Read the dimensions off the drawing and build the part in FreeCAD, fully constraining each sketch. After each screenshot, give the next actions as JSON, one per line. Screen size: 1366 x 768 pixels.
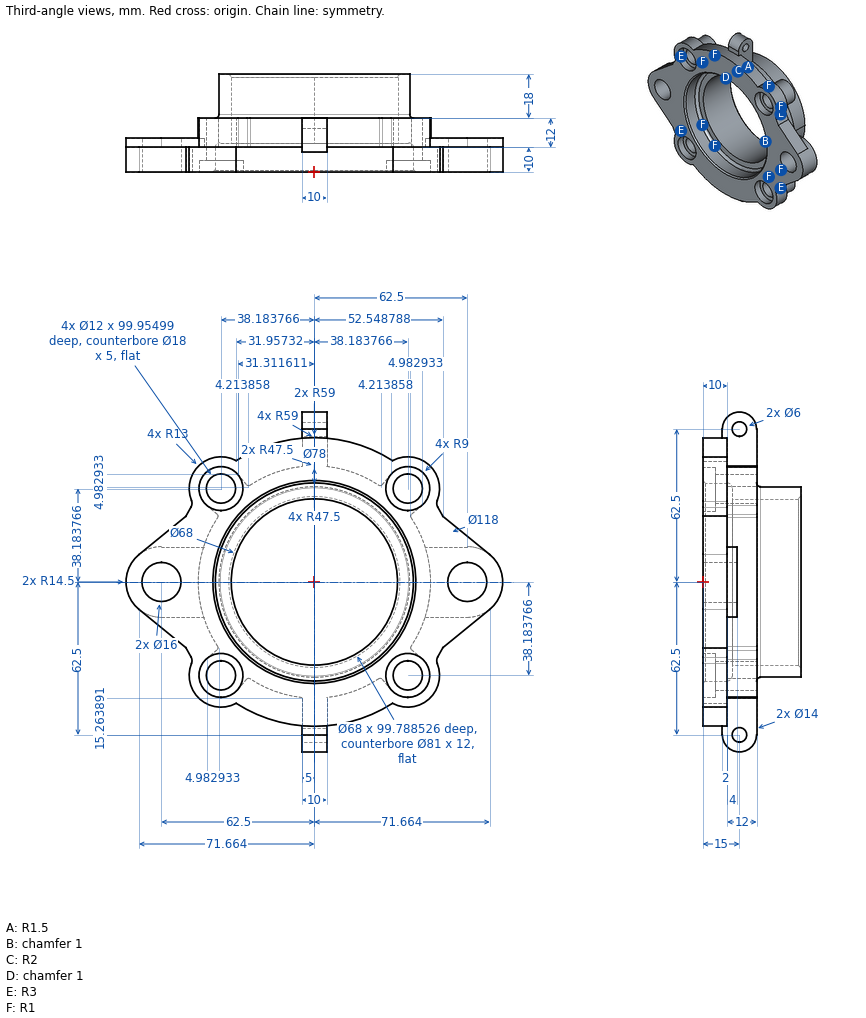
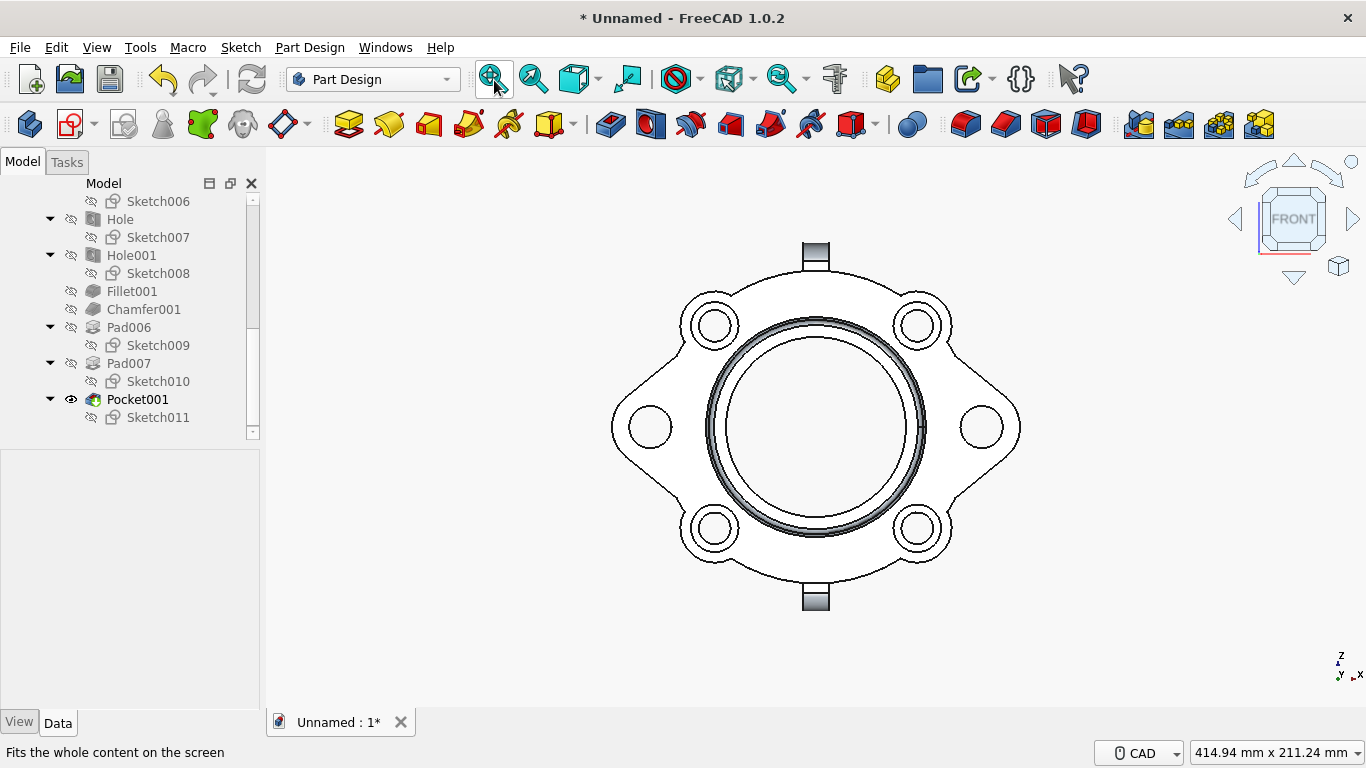
{"action": "key", "text": "3"}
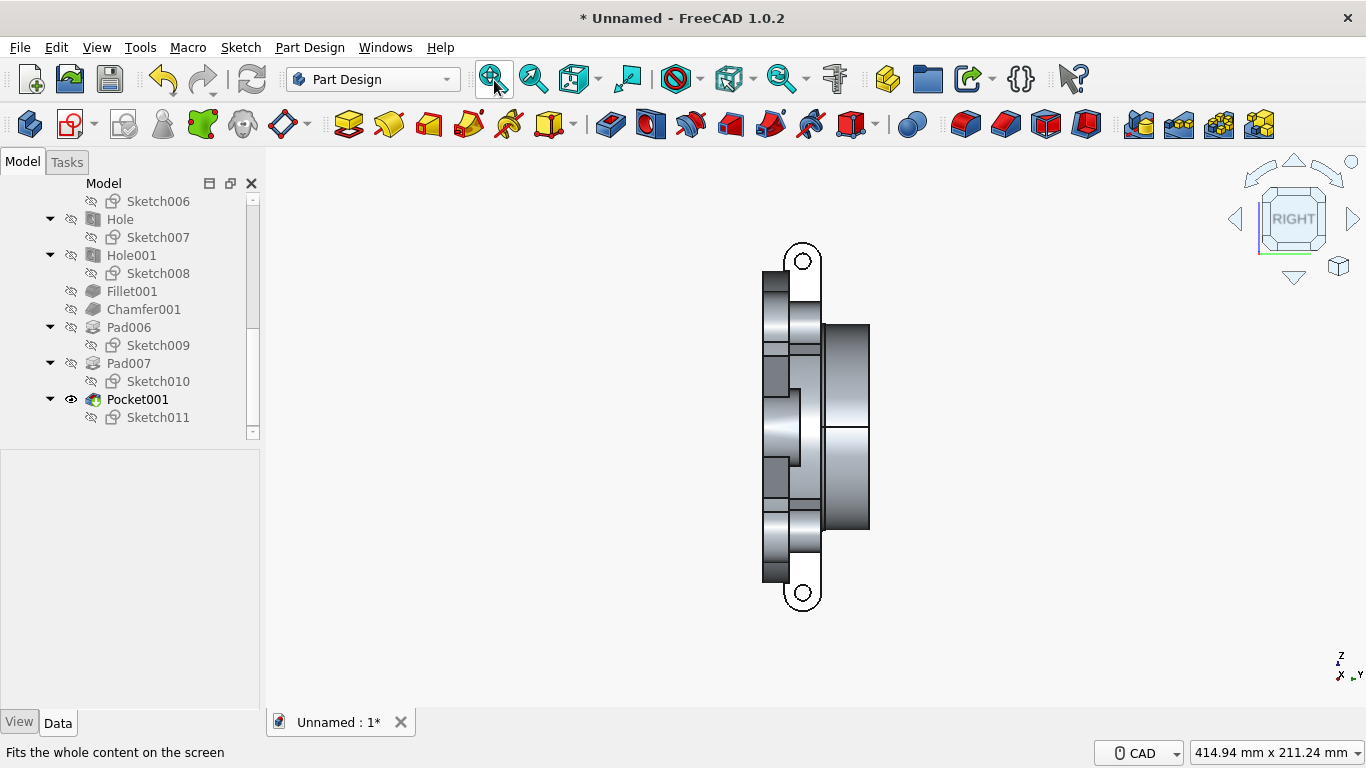
{"action": "key", "text": "5"}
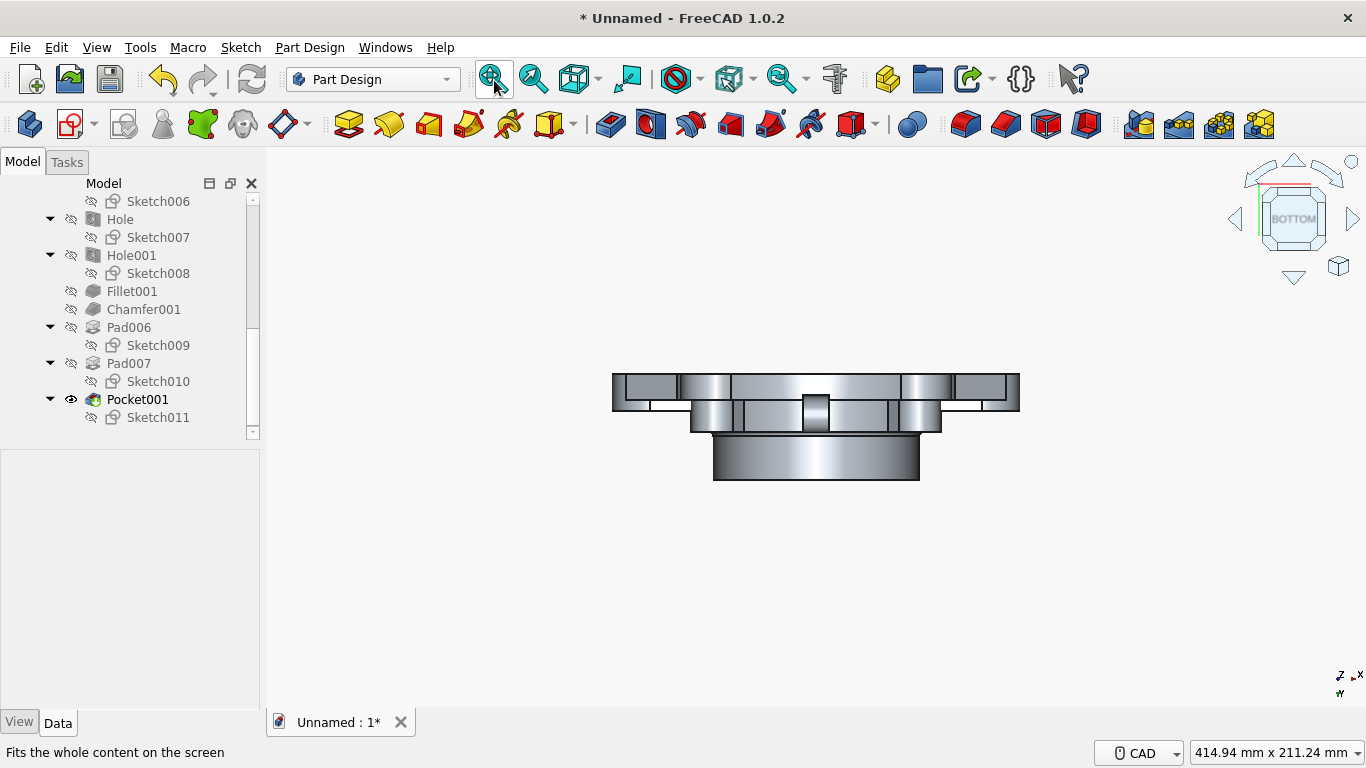
{"action": "left_click", "coordinate": [494, 80]}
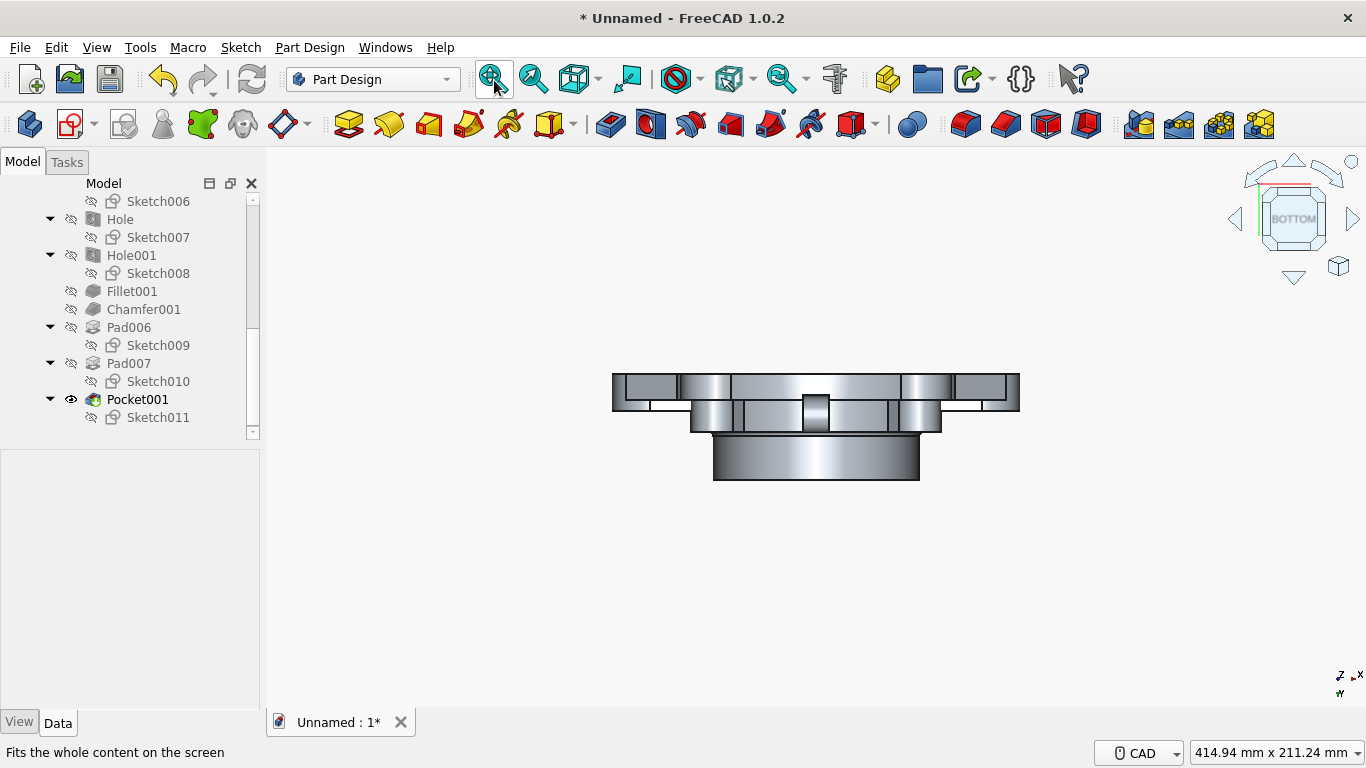
{"action": "key", "text": "4"}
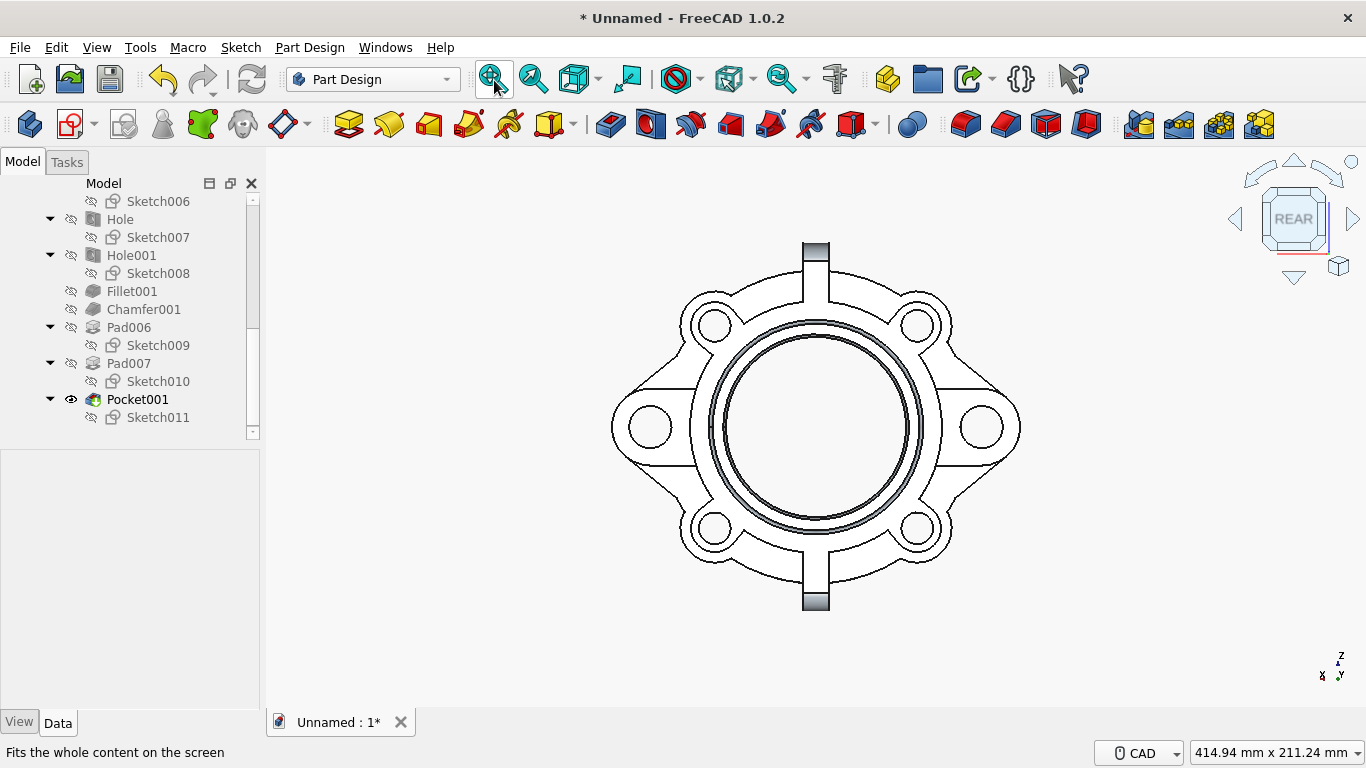
{"action": "key", "text": "6"}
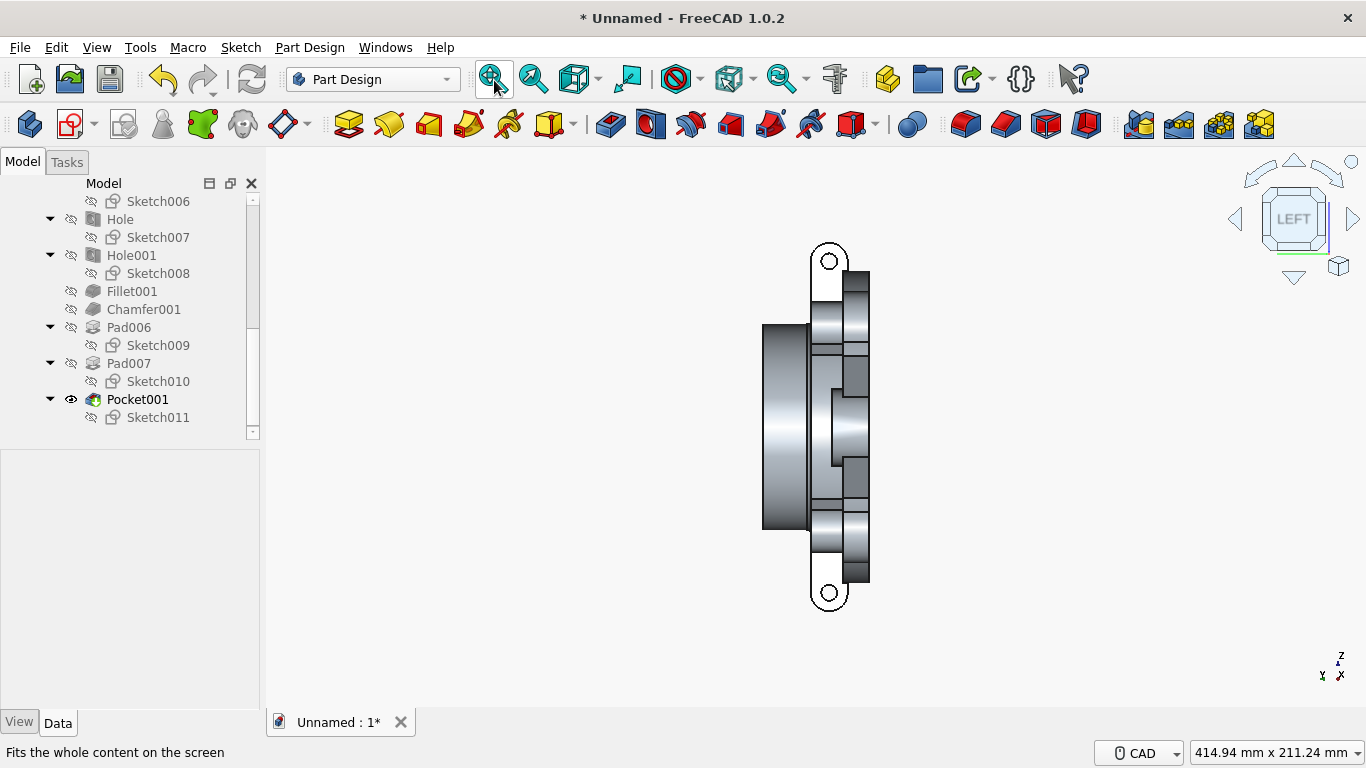
{"action": "key", "text": "v 3"}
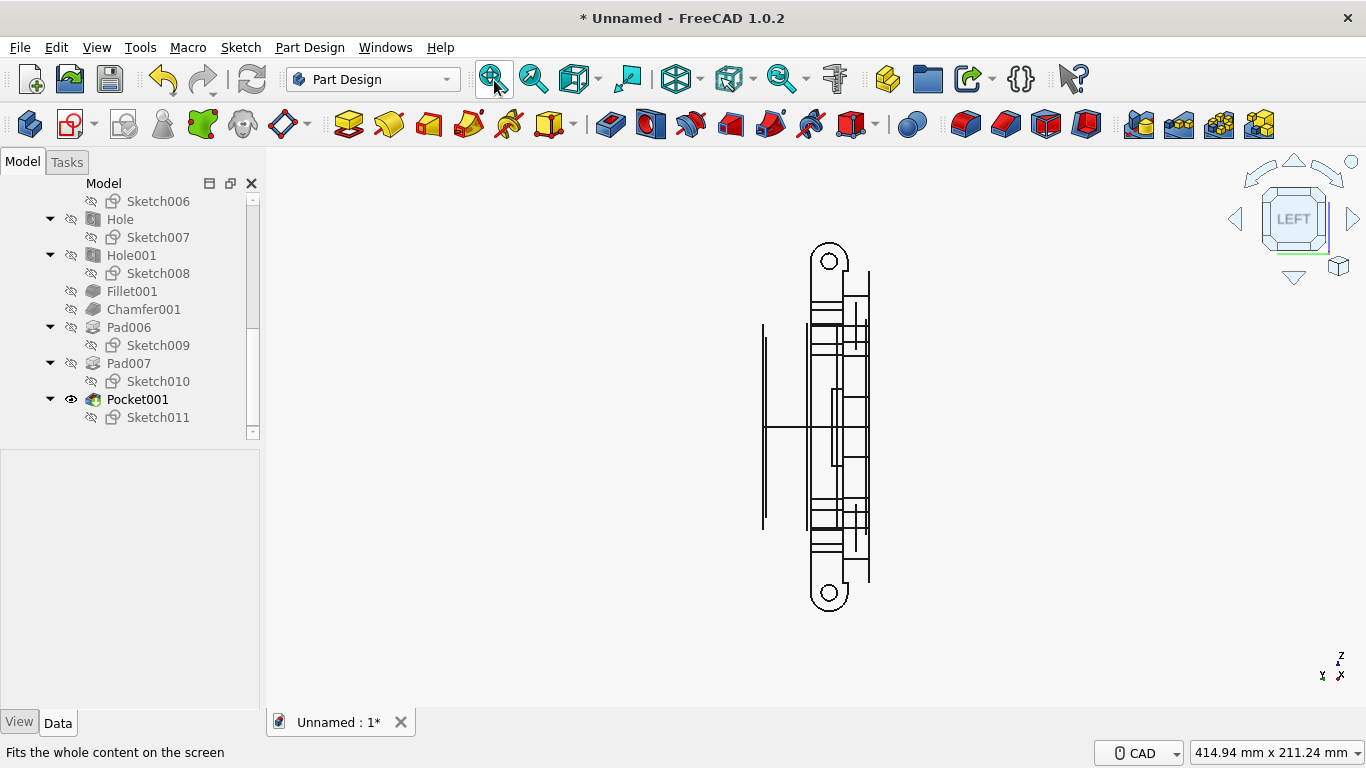
{"action": "key", "text": "0"}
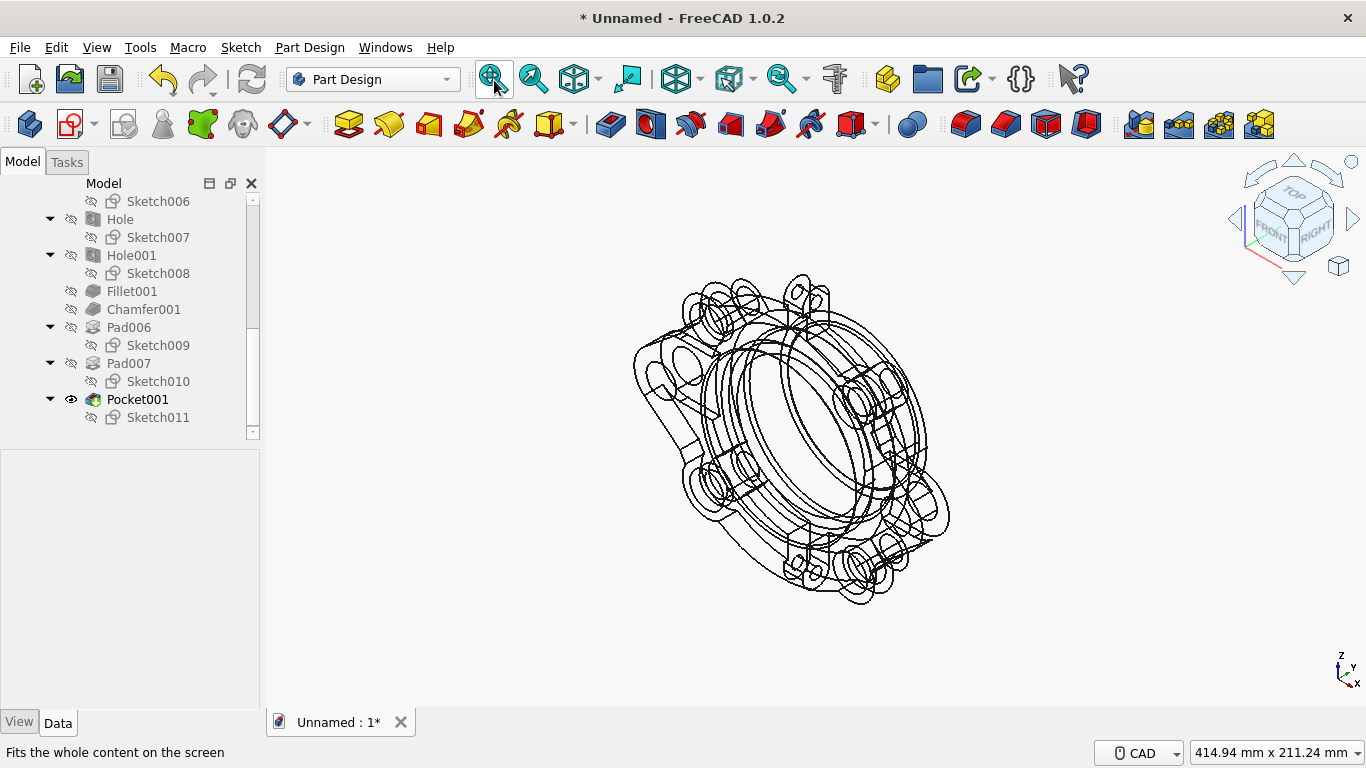
{"action": "left_click", "coordinate": [695, 458]}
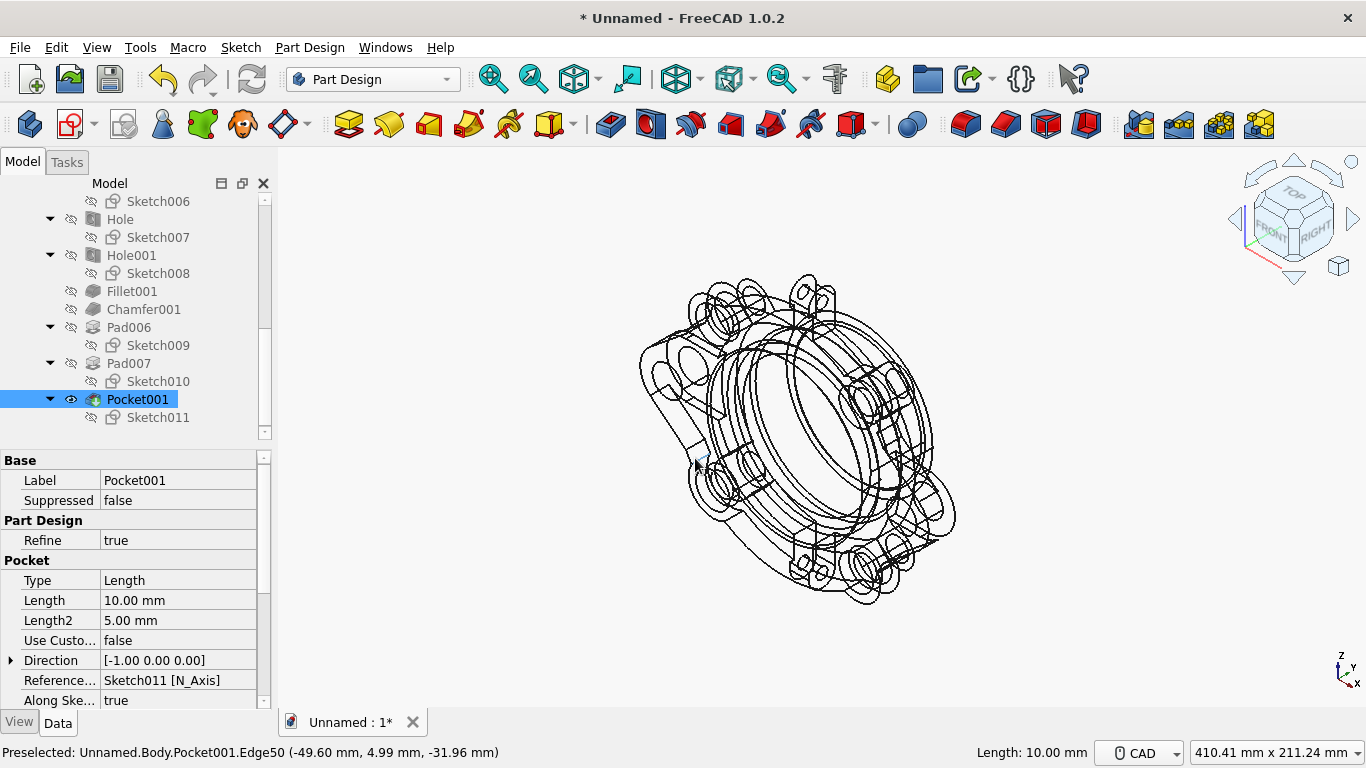
{"action": "left_click", "coordinate": [887, 427], "text": "ctrl"}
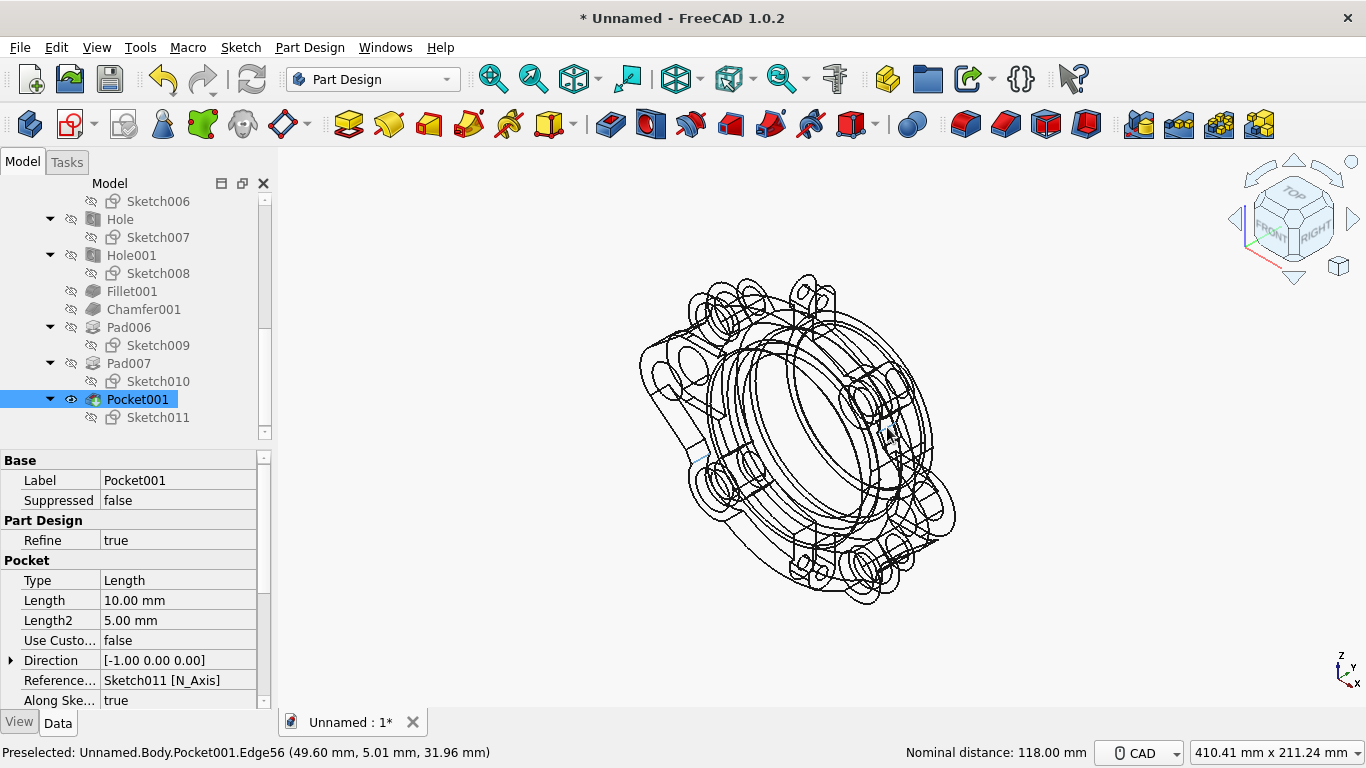
{"action": "key", "text": "2"}